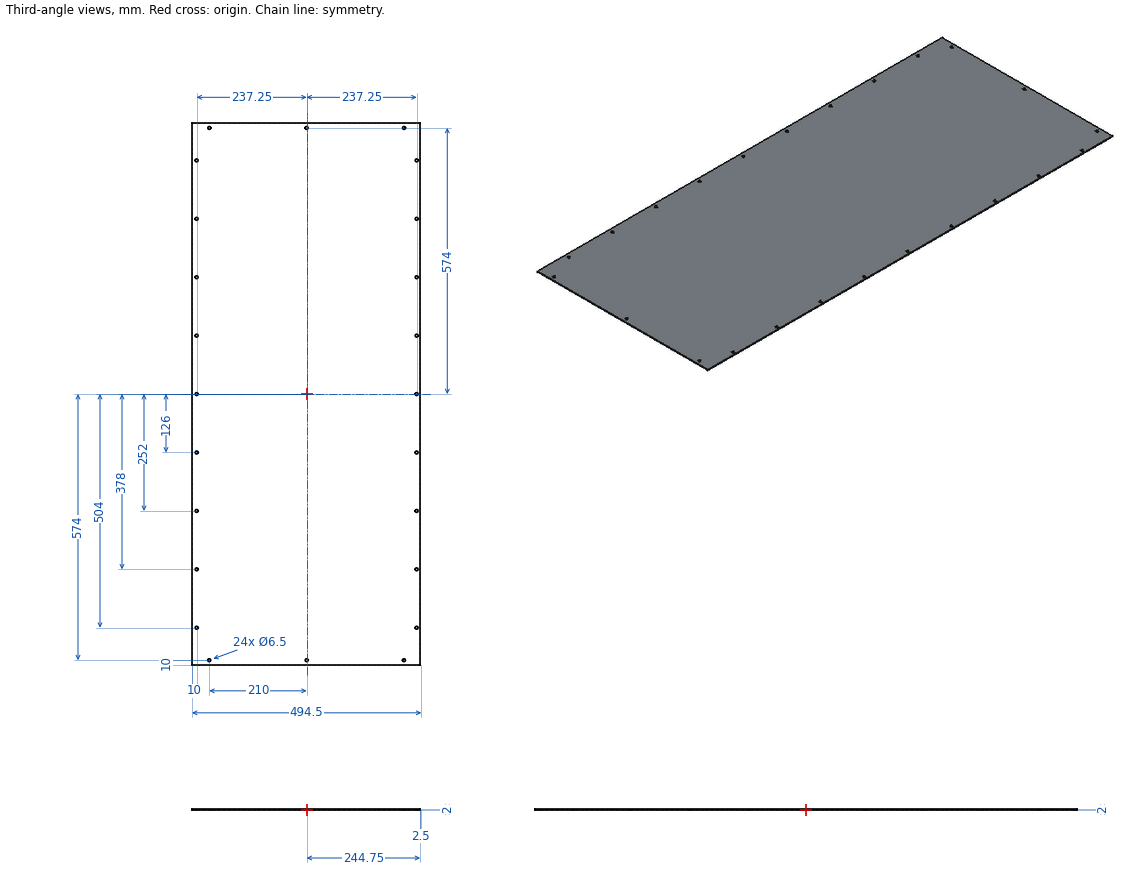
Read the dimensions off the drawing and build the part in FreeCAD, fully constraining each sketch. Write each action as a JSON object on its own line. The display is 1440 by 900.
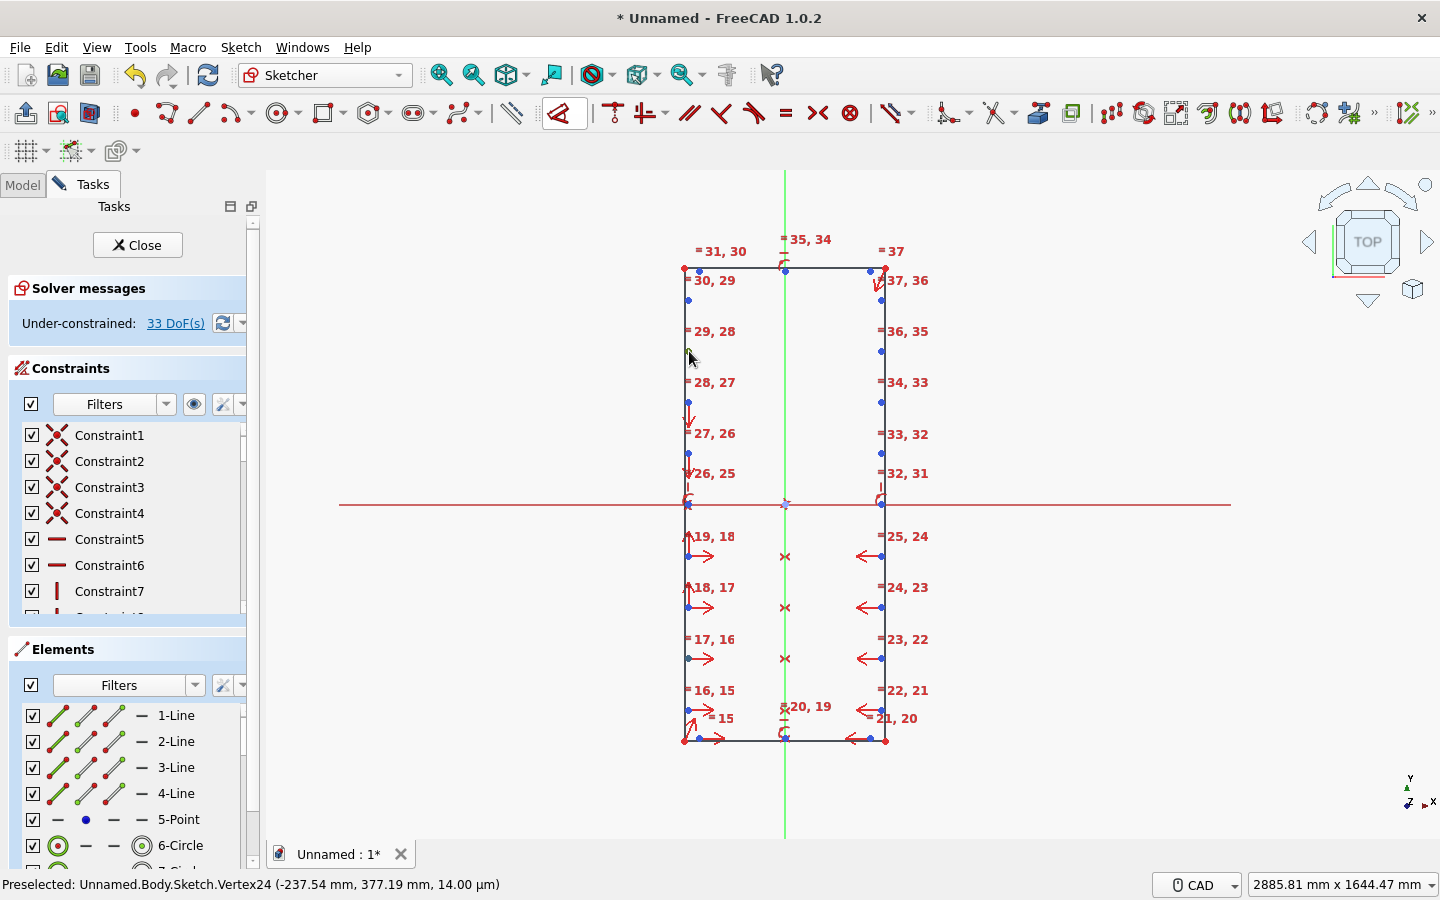
{"action": "left_click", "coordinate": [364, 505]}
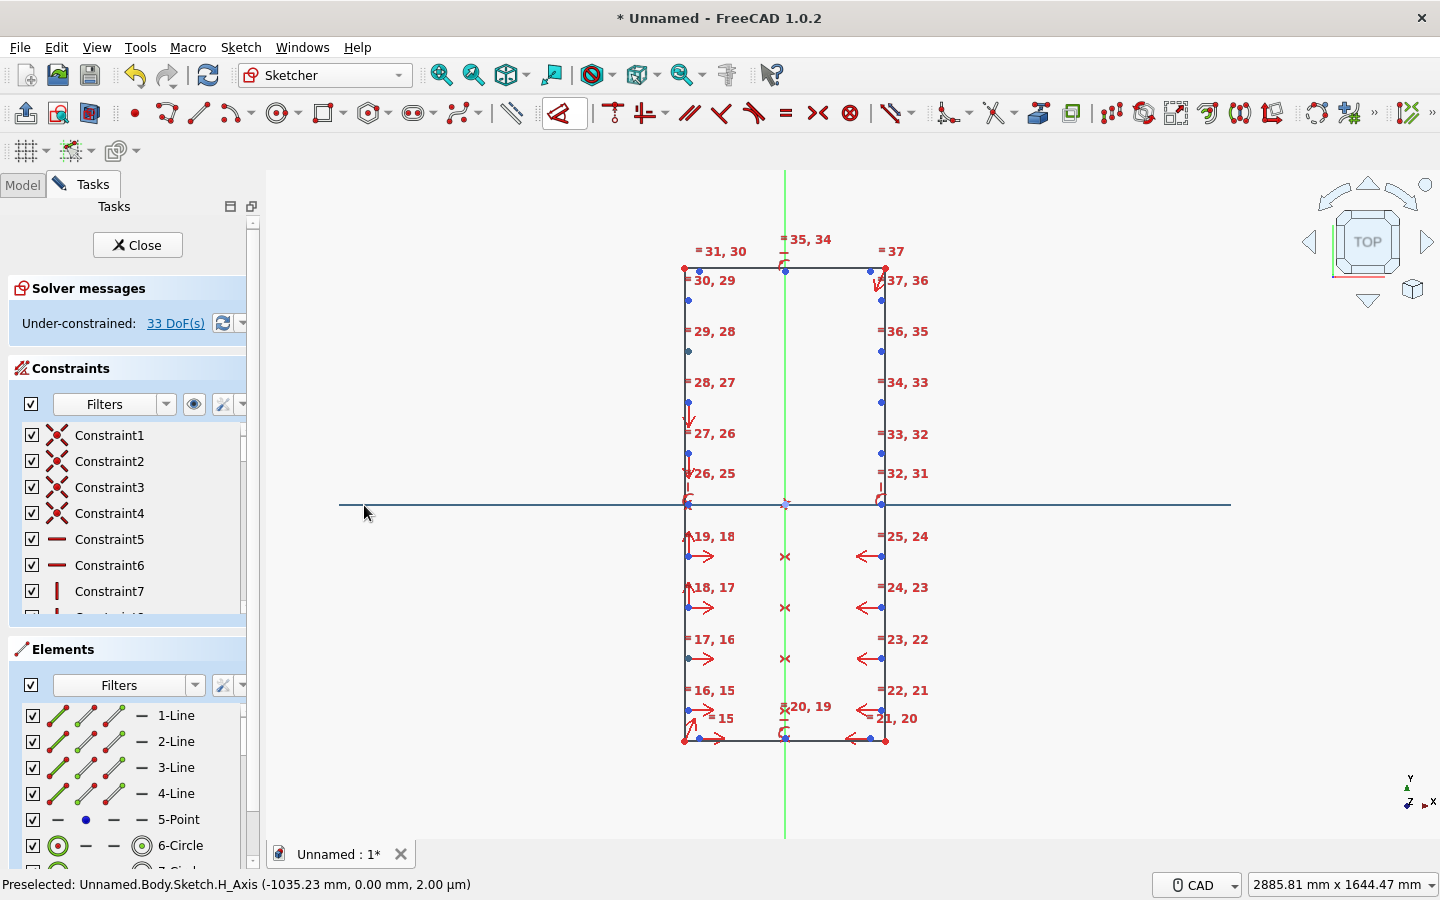
{"action": "left_click", "coordinate": [818, 114]}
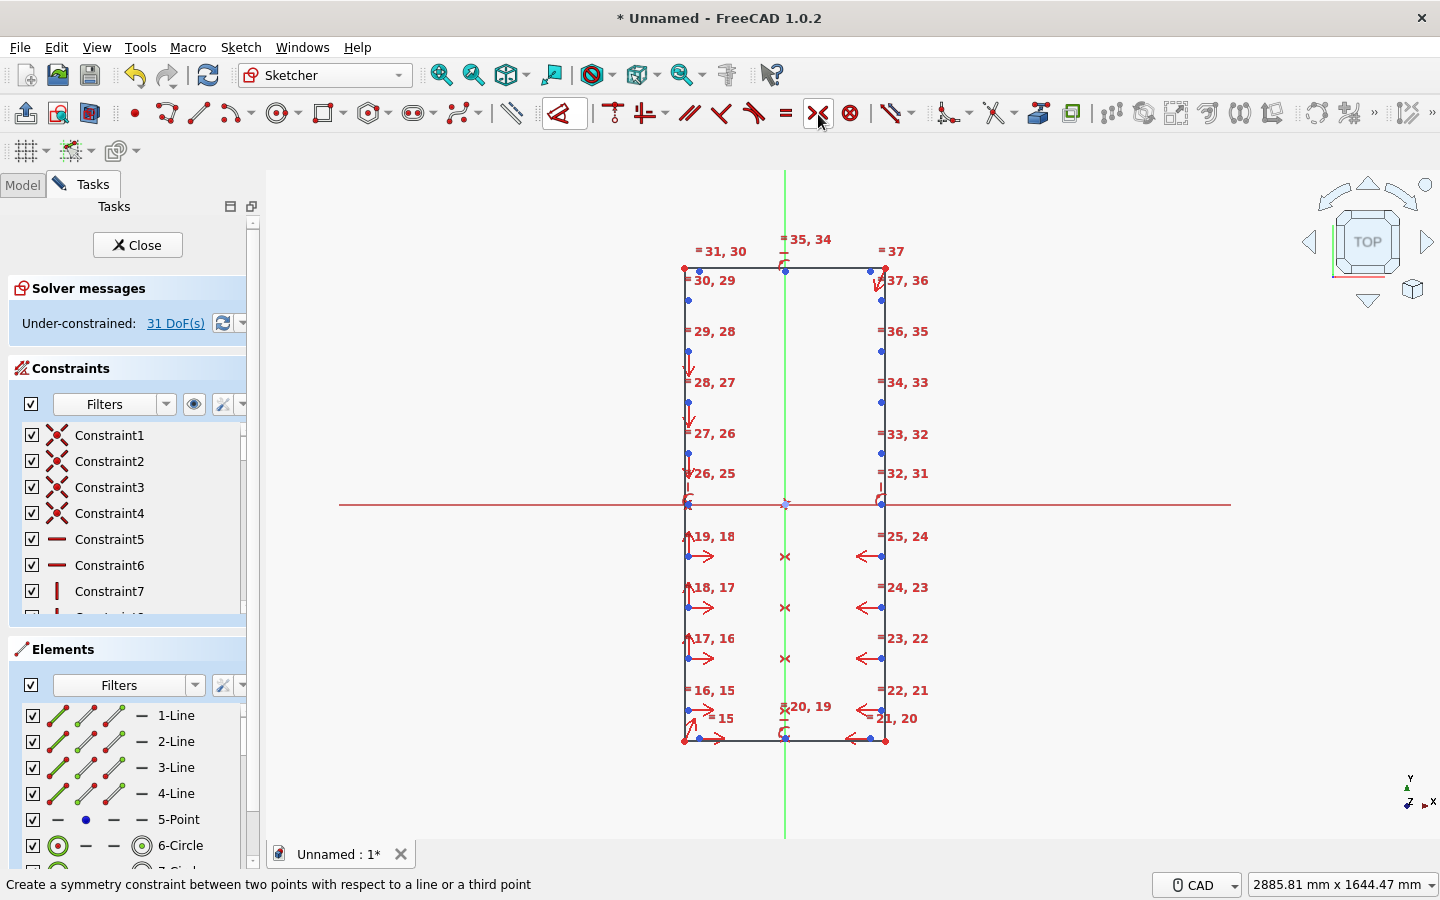
{"action": "left_click", "coordinate": [689, 710]}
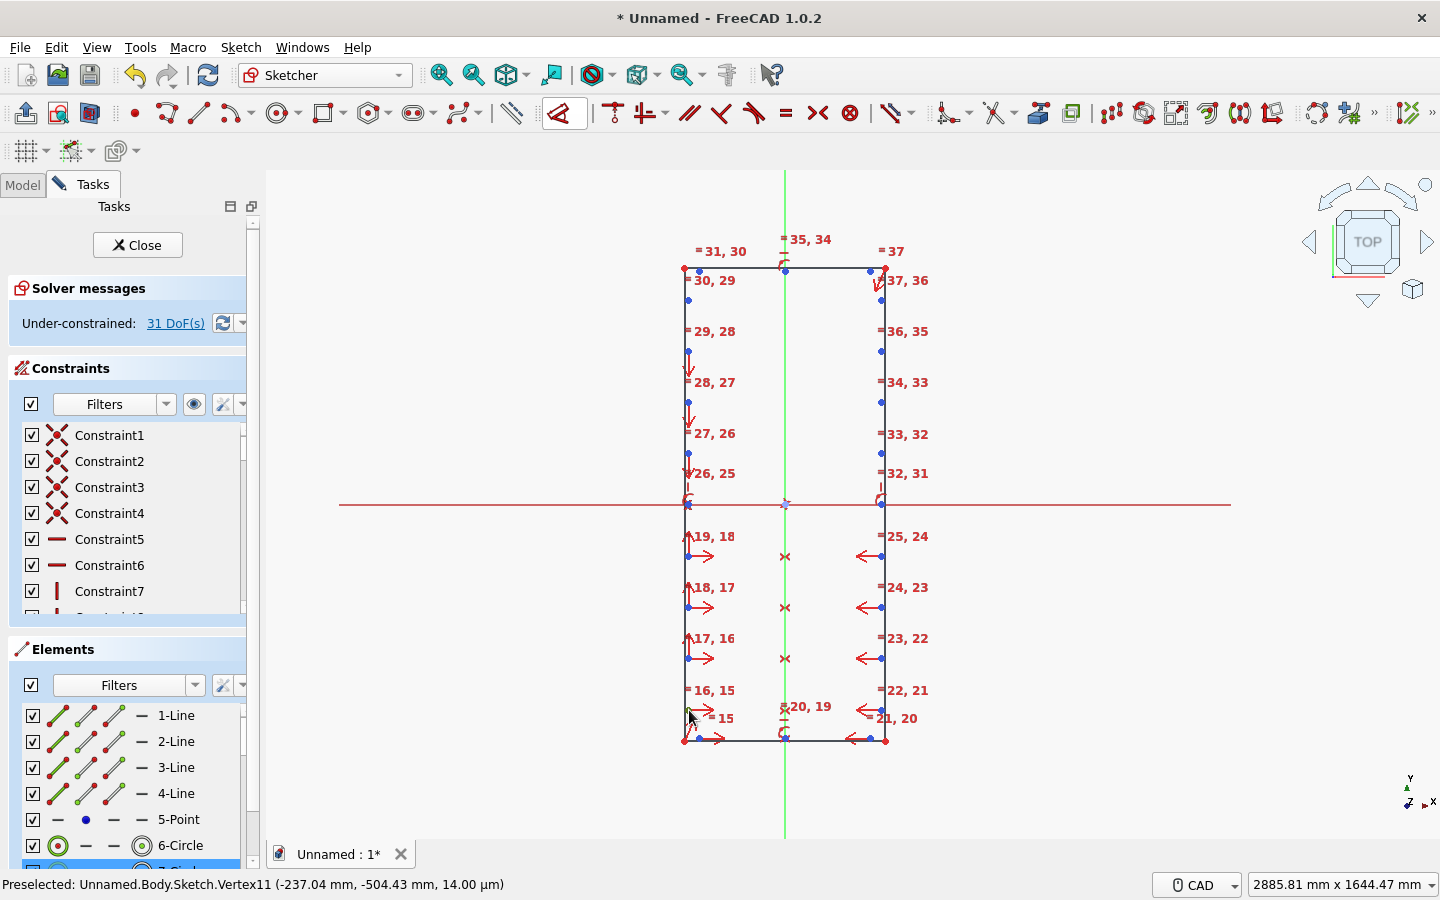
{"action": "left_click", "coordinate": [689, 300]}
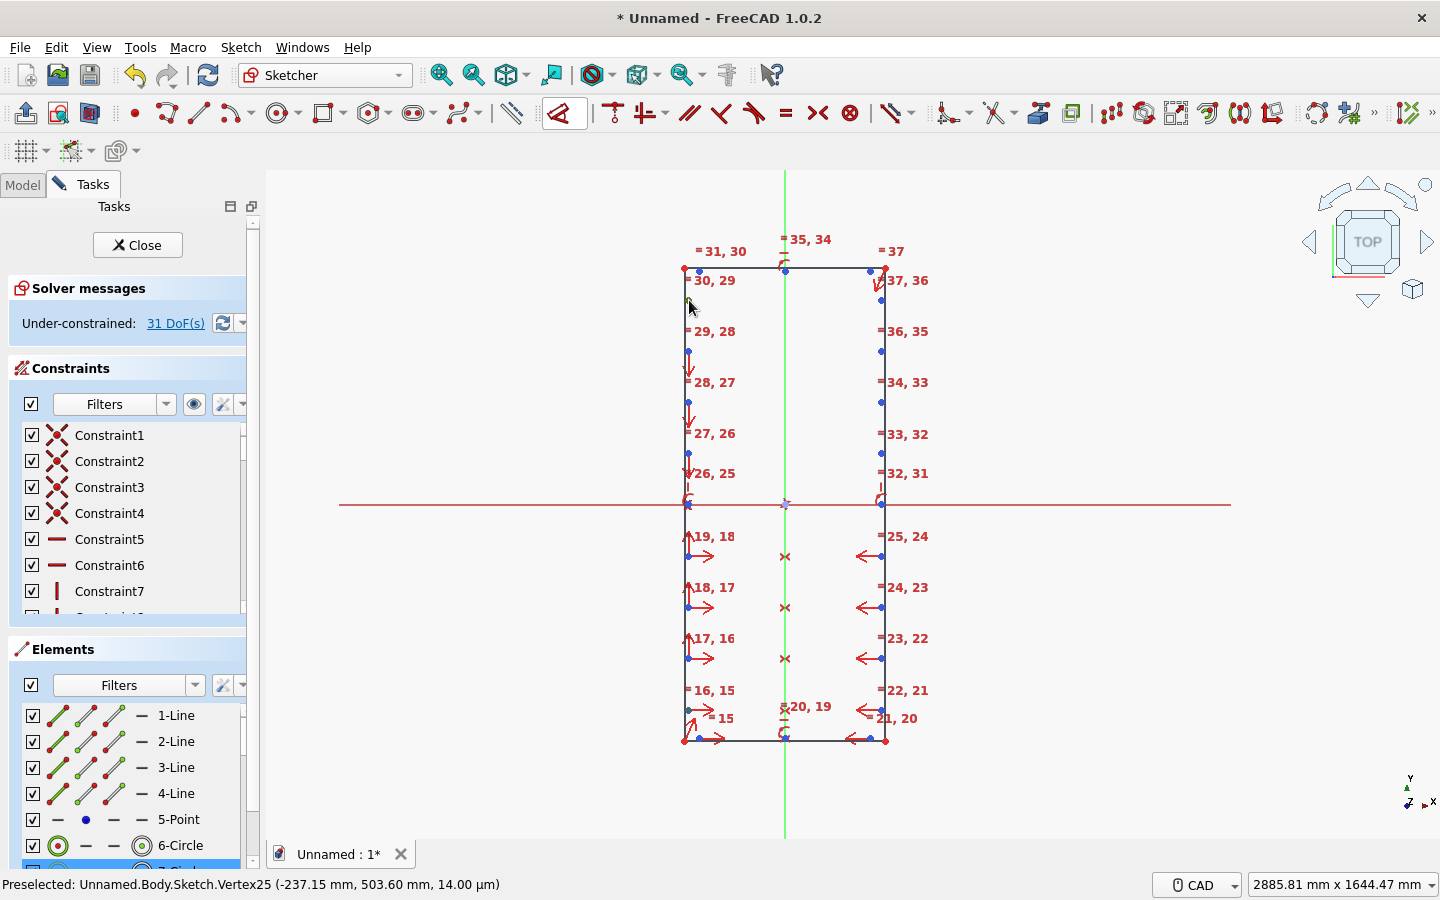
{"action": "left_click", "coordinate": [364, 505]}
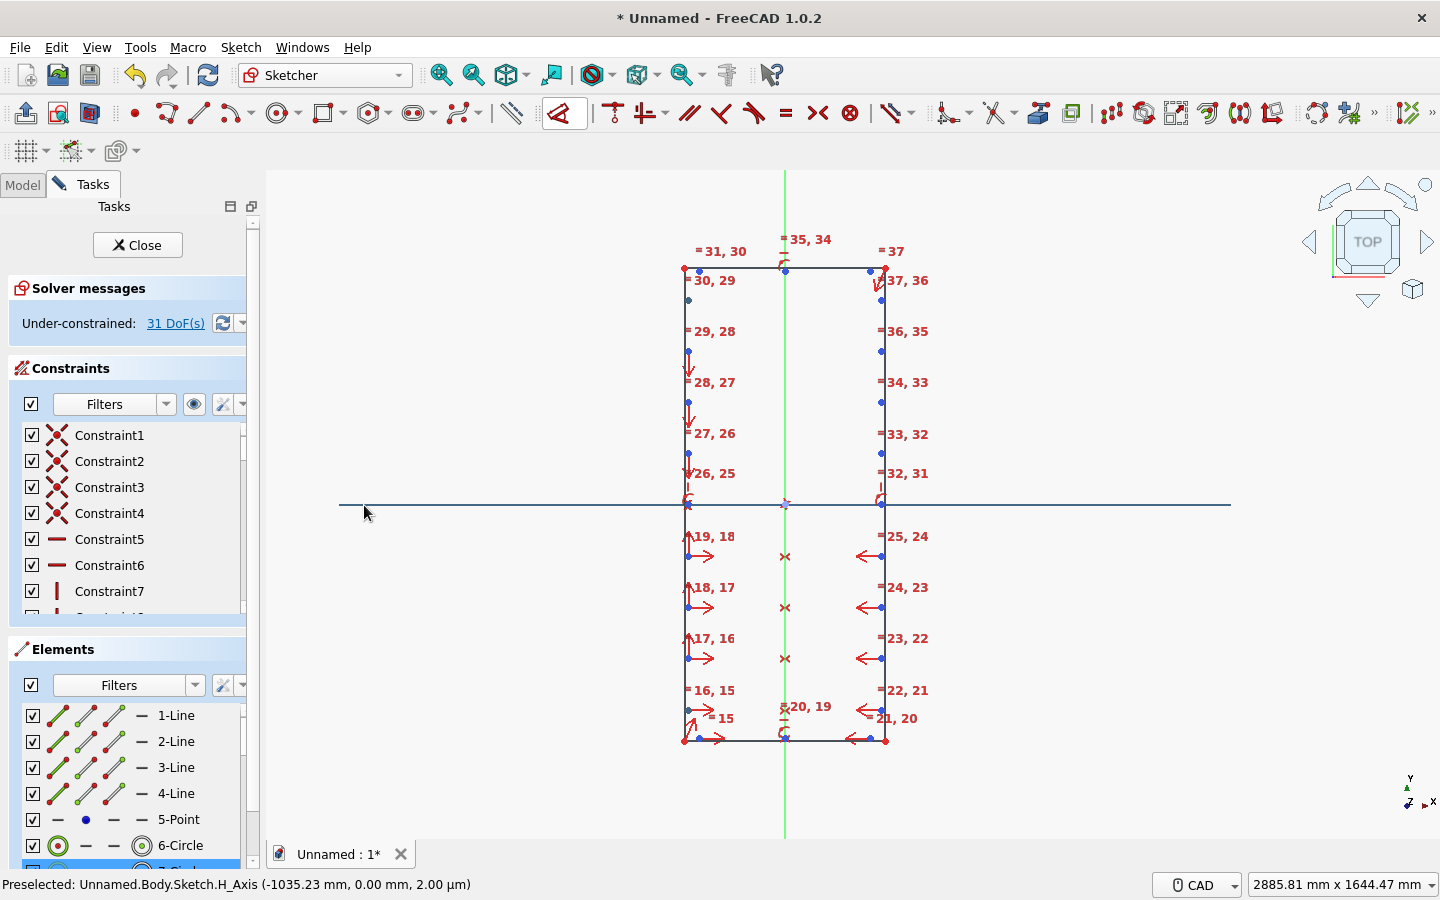
{"action": "left_click", "coordinate": [818, 114]}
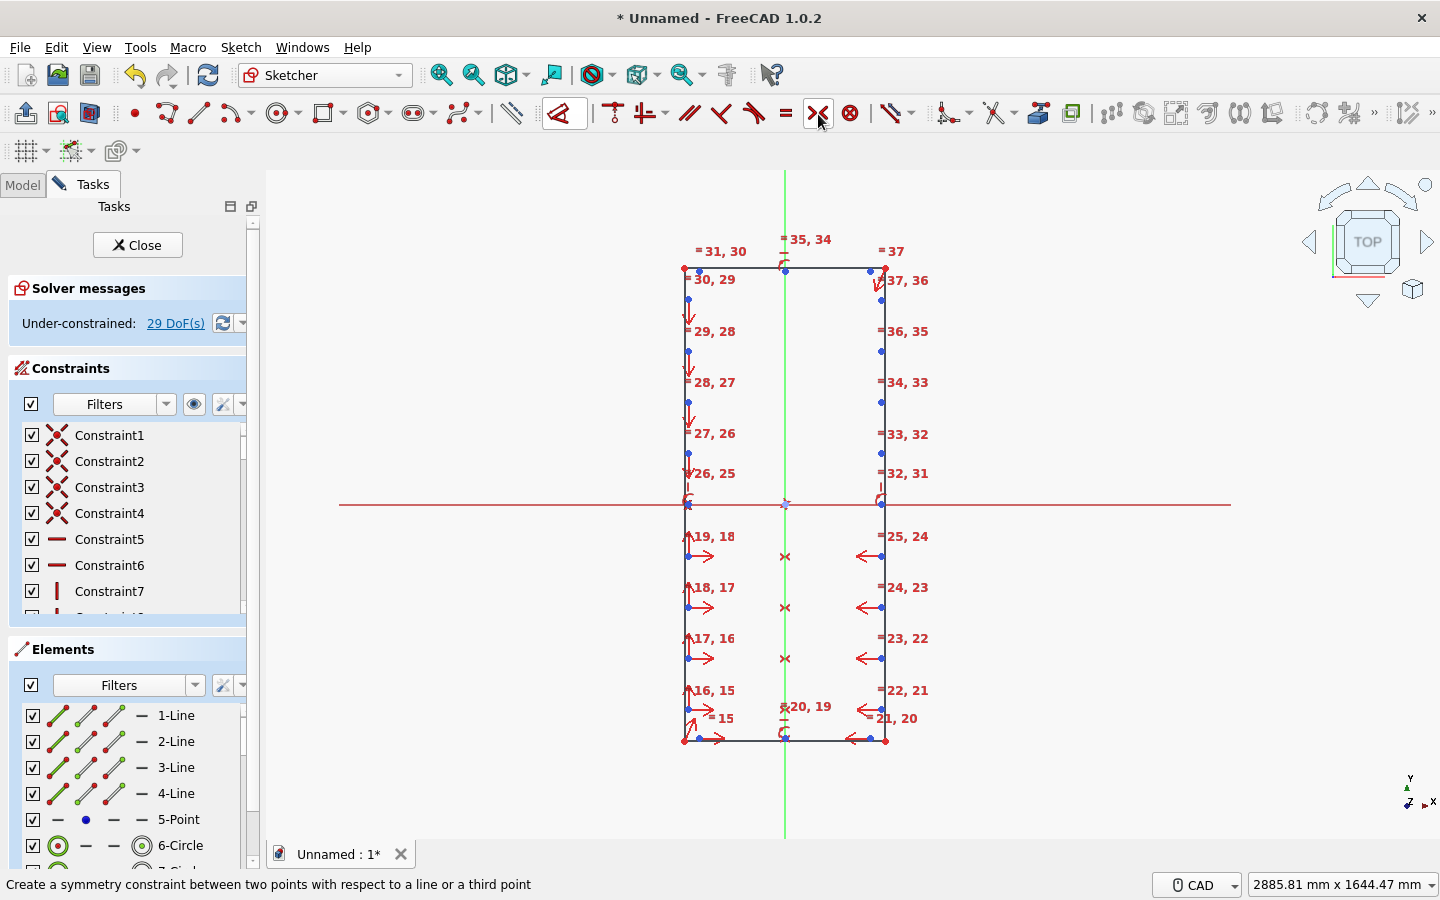
{"action": "left_click", "coordinate": [700, 739]}